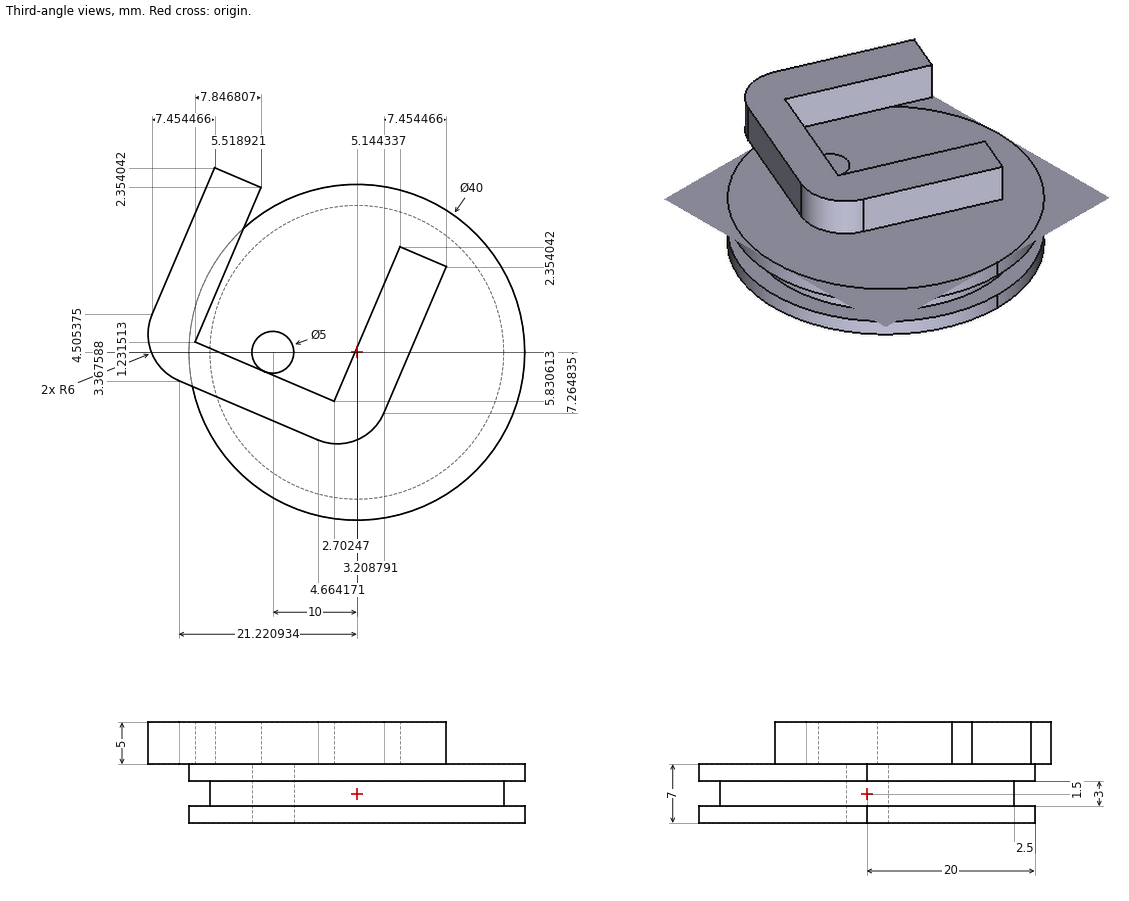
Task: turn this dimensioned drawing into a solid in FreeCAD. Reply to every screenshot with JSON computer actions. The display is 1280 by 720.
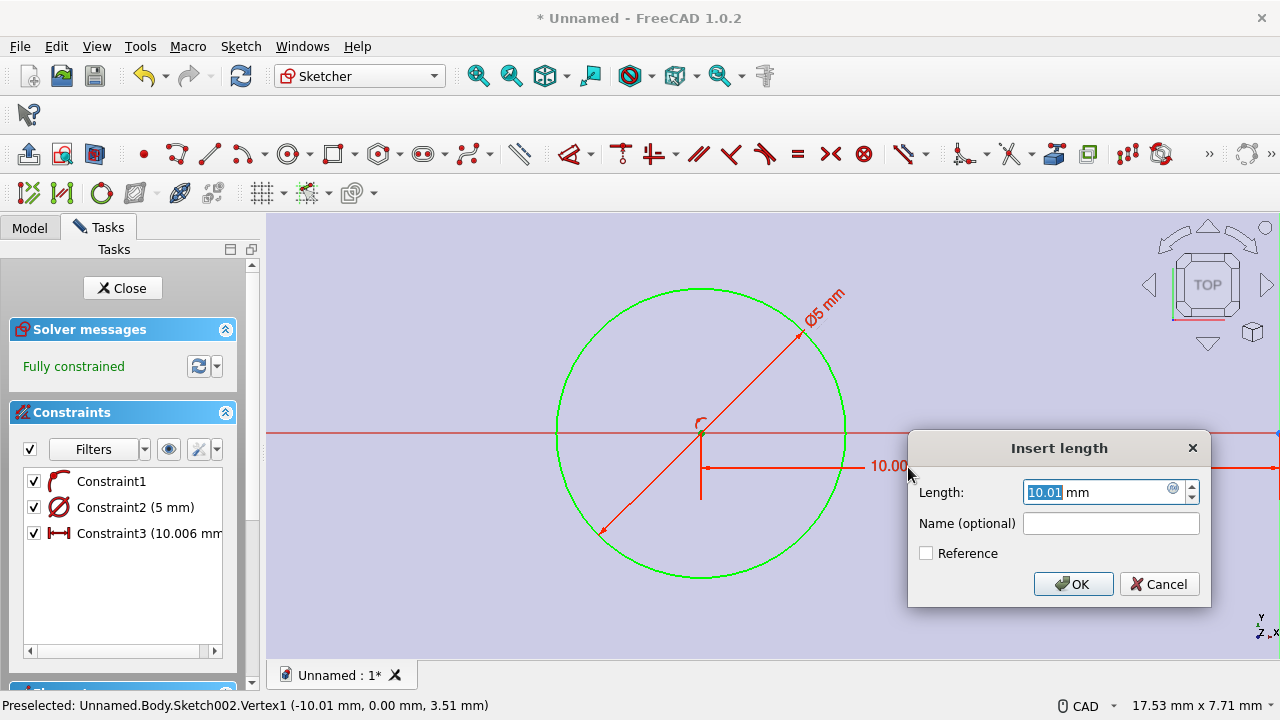
{"action": "type", "text": "10"}
{"action": "key", "text": "Return"}
{"action": "key", "text": "Escape"}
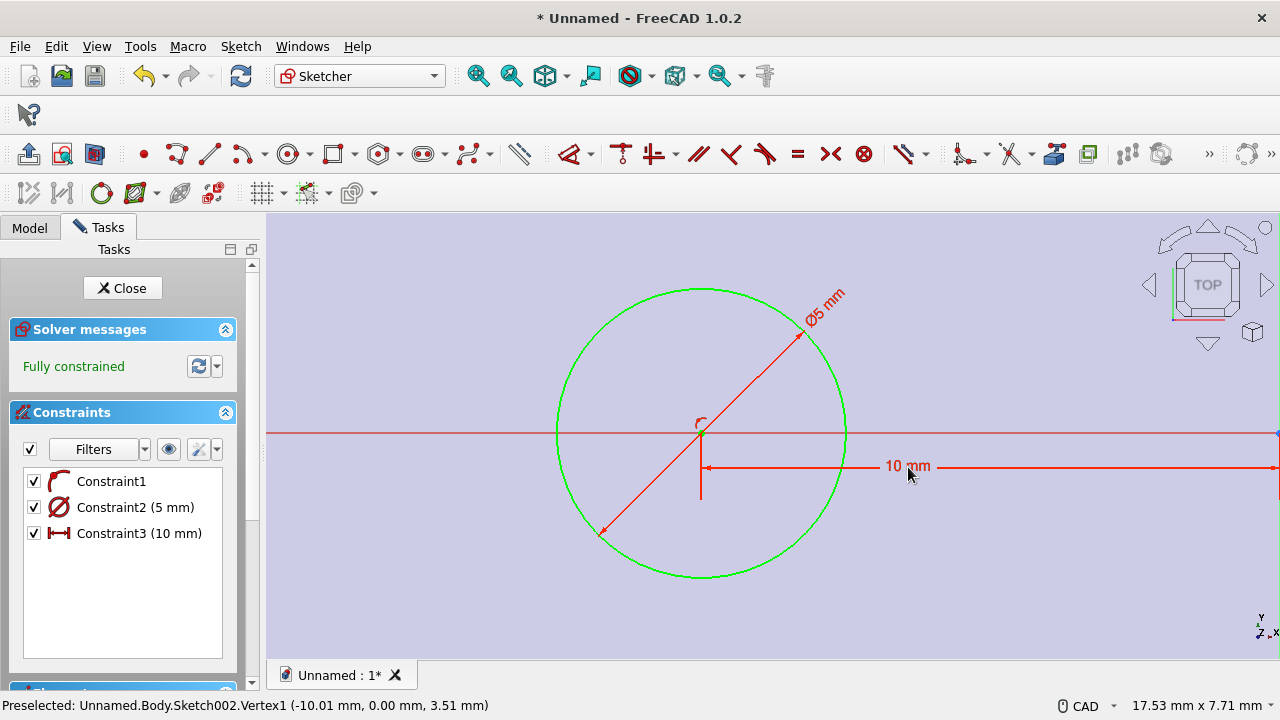
{"action": "left_click", "coordinate": [123, 288]}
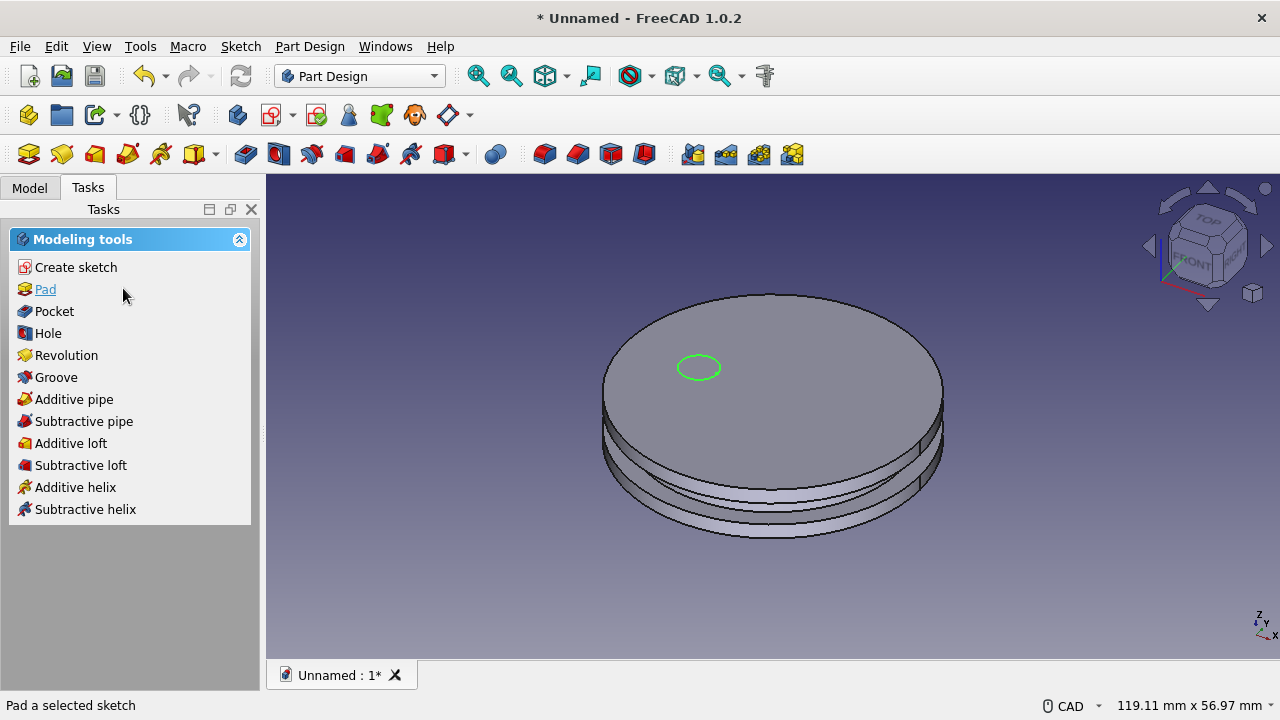
{"action": "left_click", "coordinate": [246, 154]}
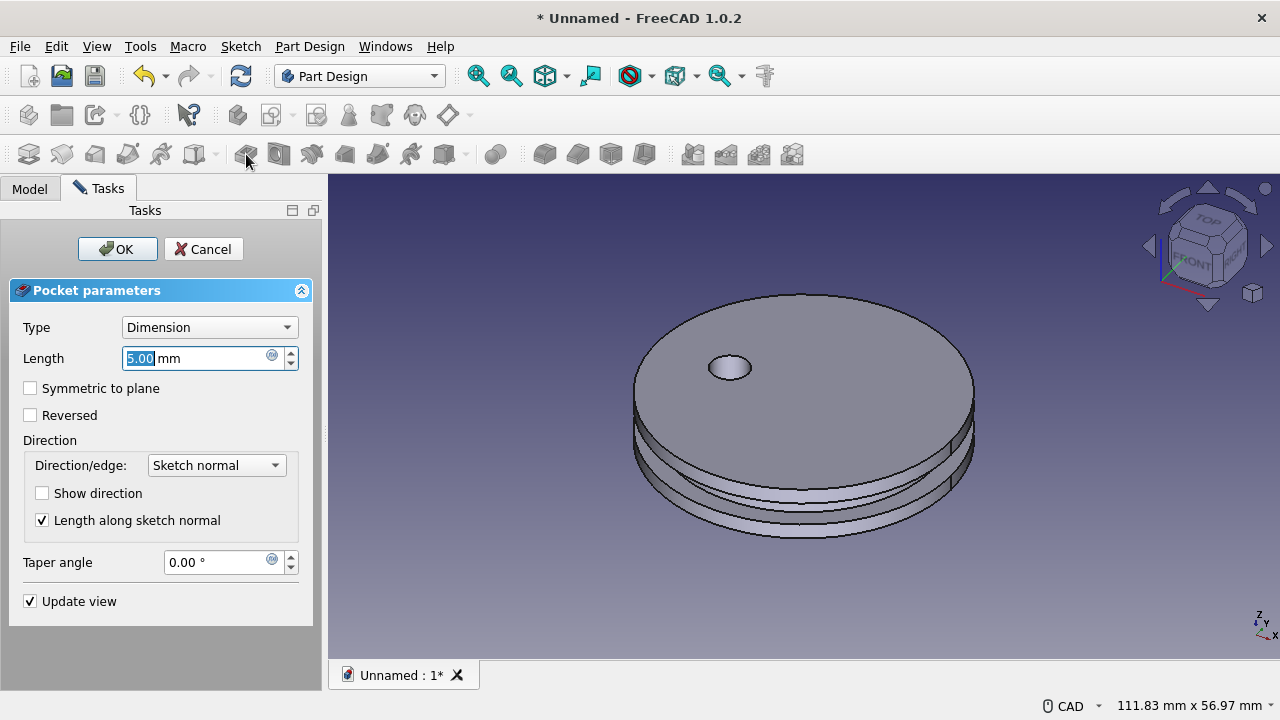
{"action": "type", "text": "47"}
{"action": "key", "text": "Tab"}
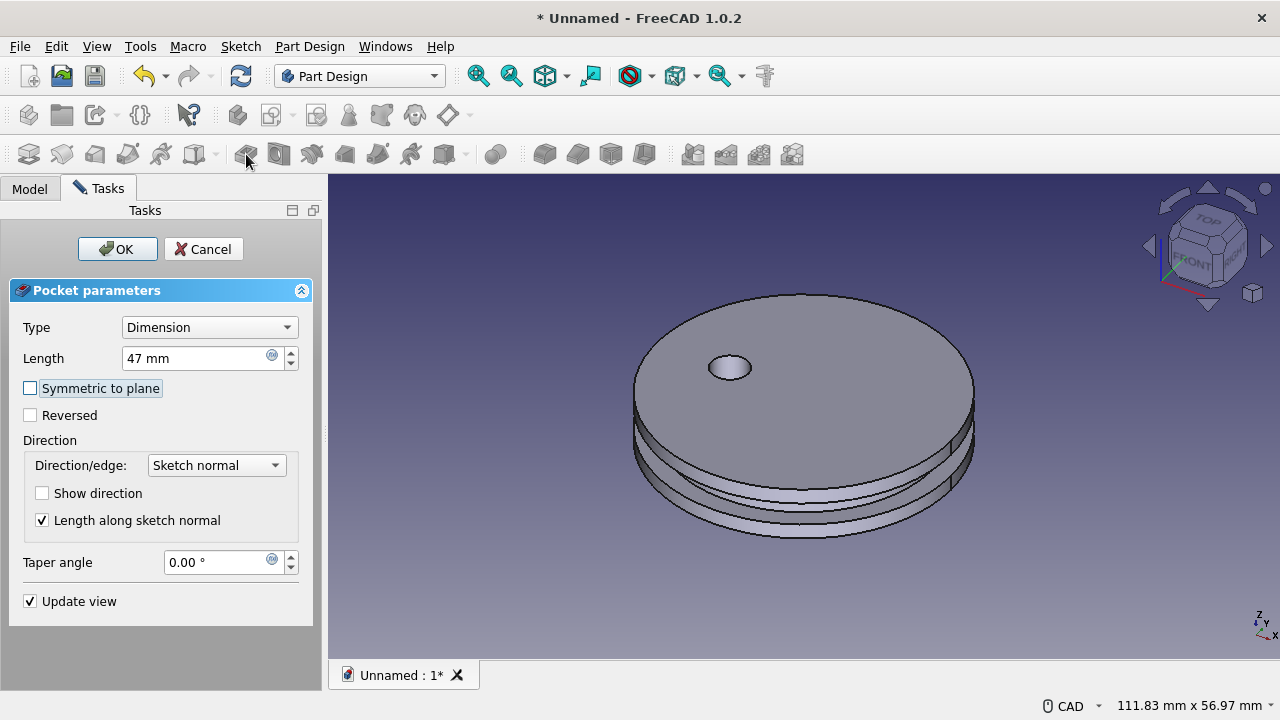
{"action": "left_click", "coordinate": [118, 249]}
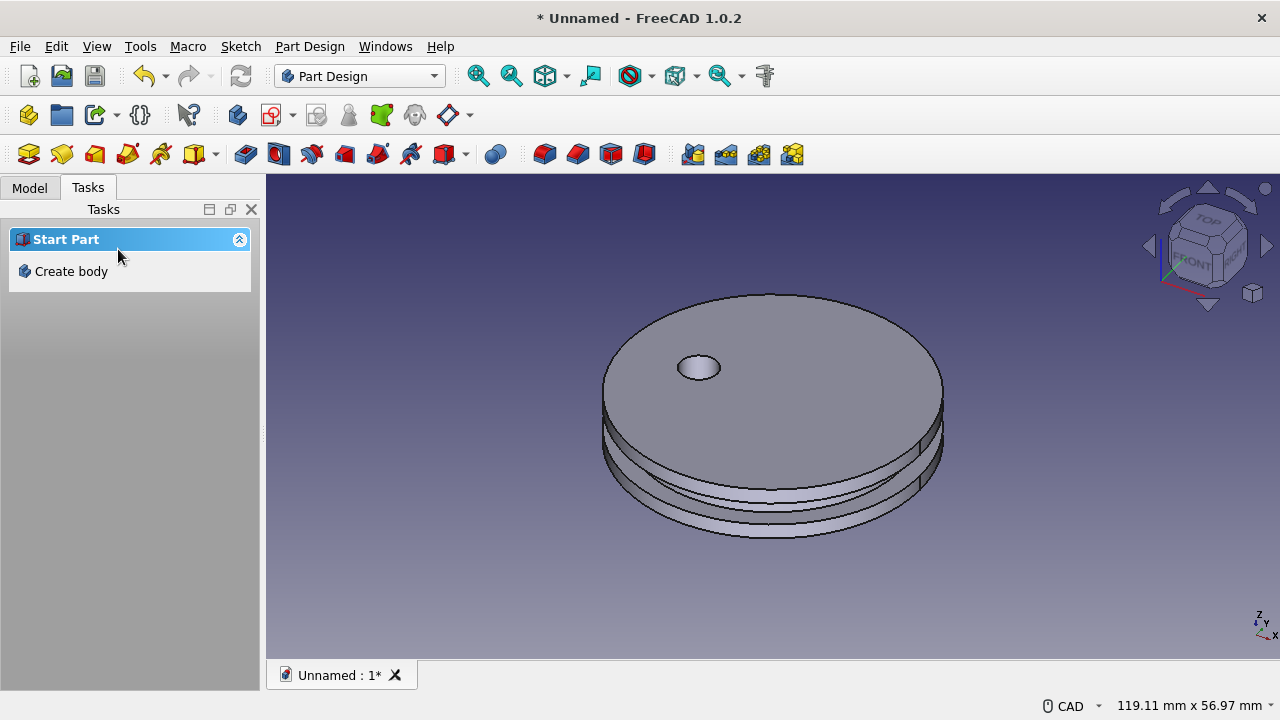
{"action": "left_click", "coordinate": [815, 405]}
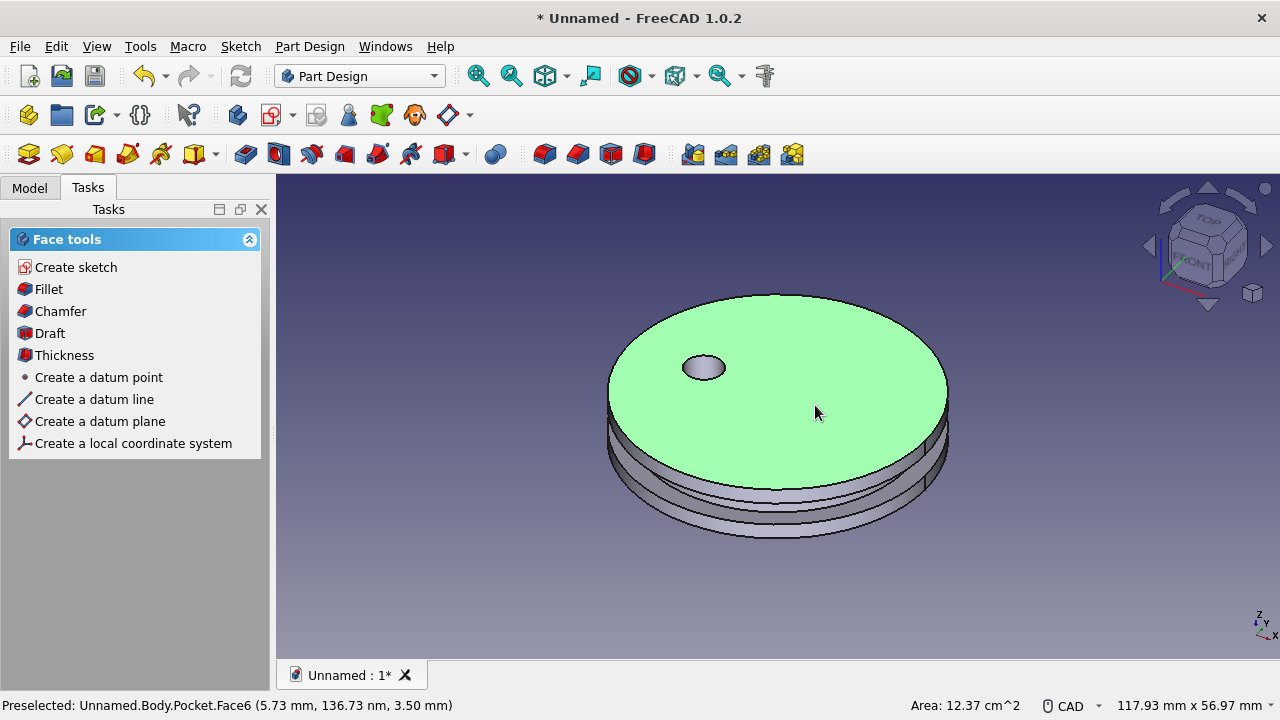
{"action": "left_click", "coordinate": [270, 116]}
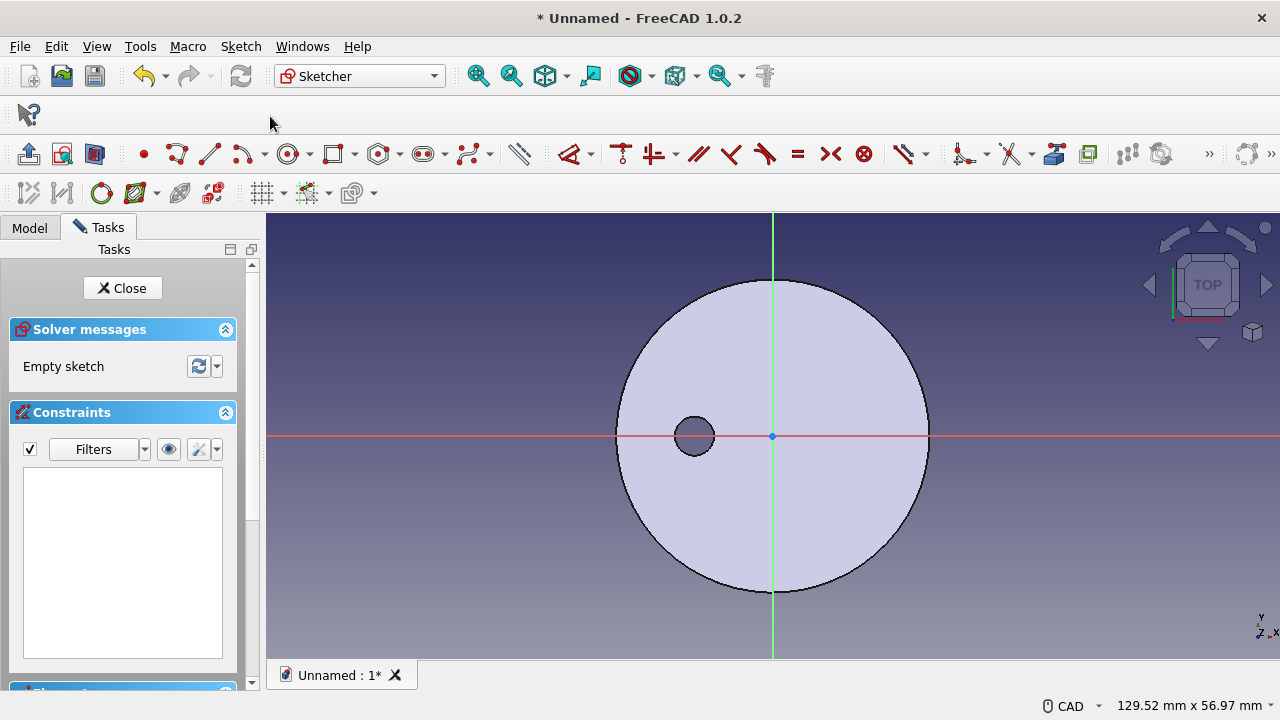
{"action": "scroll", "coordinate": [640, 631], "scroll_direction": "down", "scroll_amount": 1}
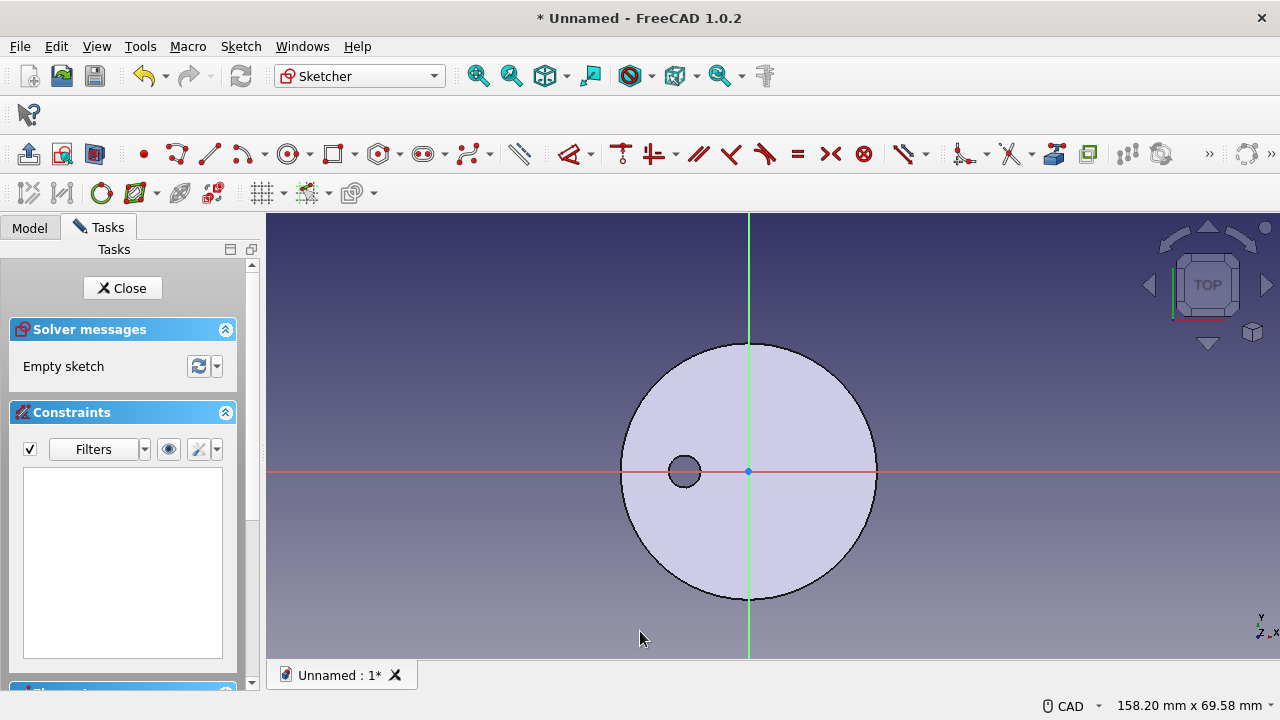
{"action": "left_click", "coordinate": [210, 154]}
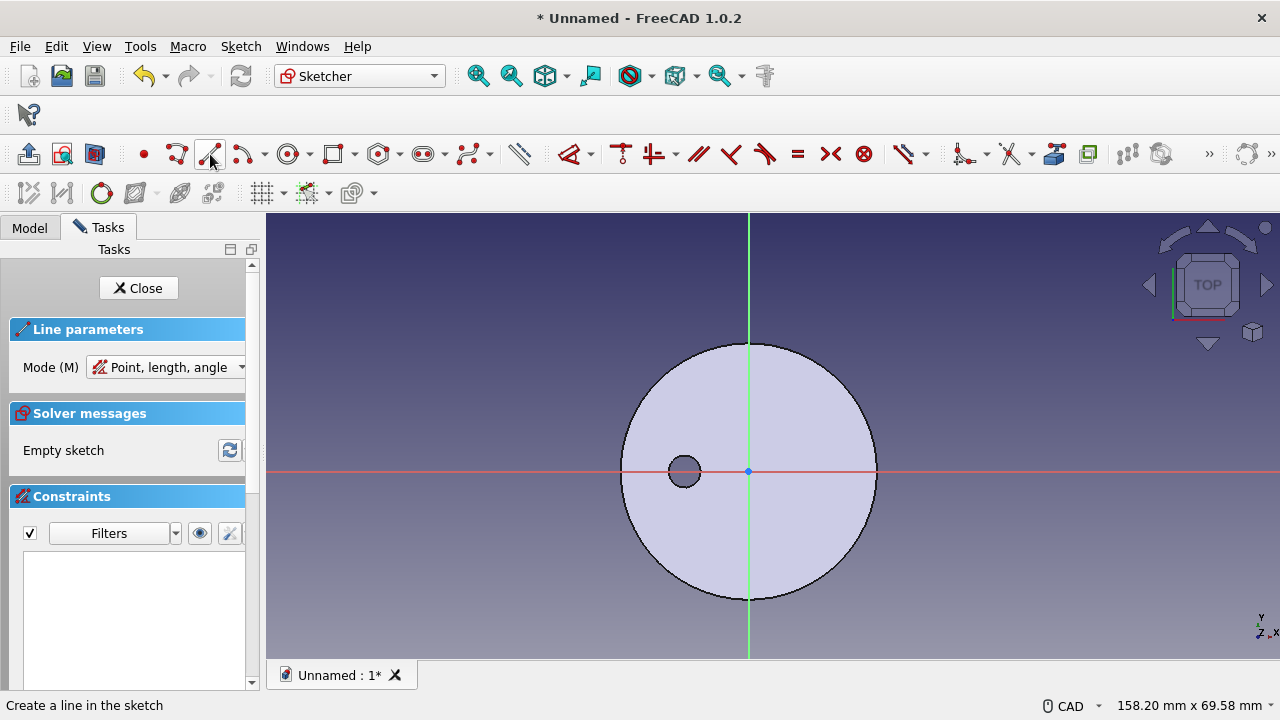
{"action": "left_click", "coordinate": [613, 493]}
{"action": "left_click", "coordinate": [719, 538]}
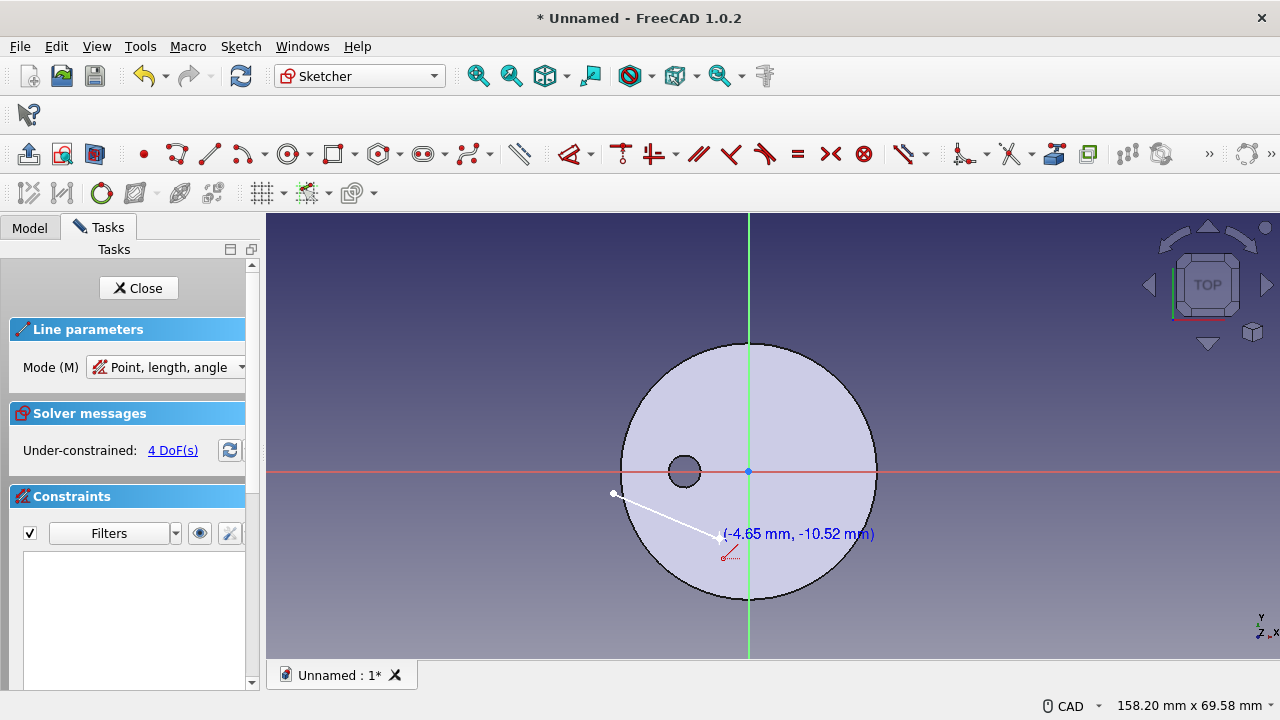
{"action": "left_click", "coordinate": [177, 154]}